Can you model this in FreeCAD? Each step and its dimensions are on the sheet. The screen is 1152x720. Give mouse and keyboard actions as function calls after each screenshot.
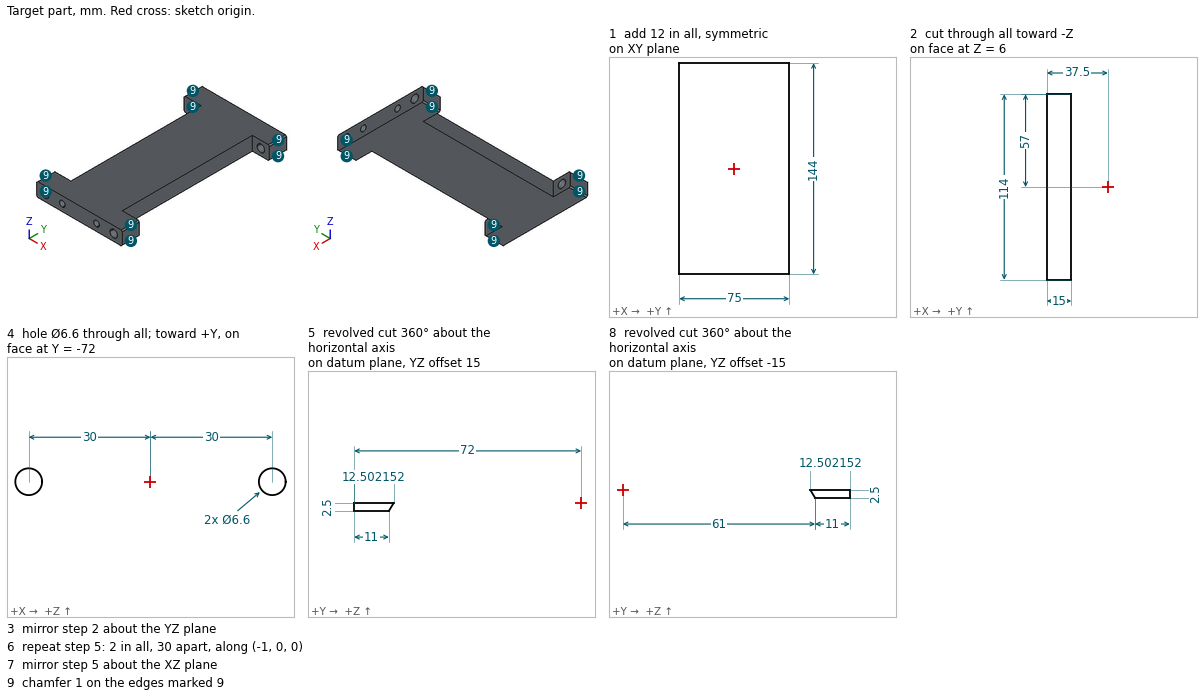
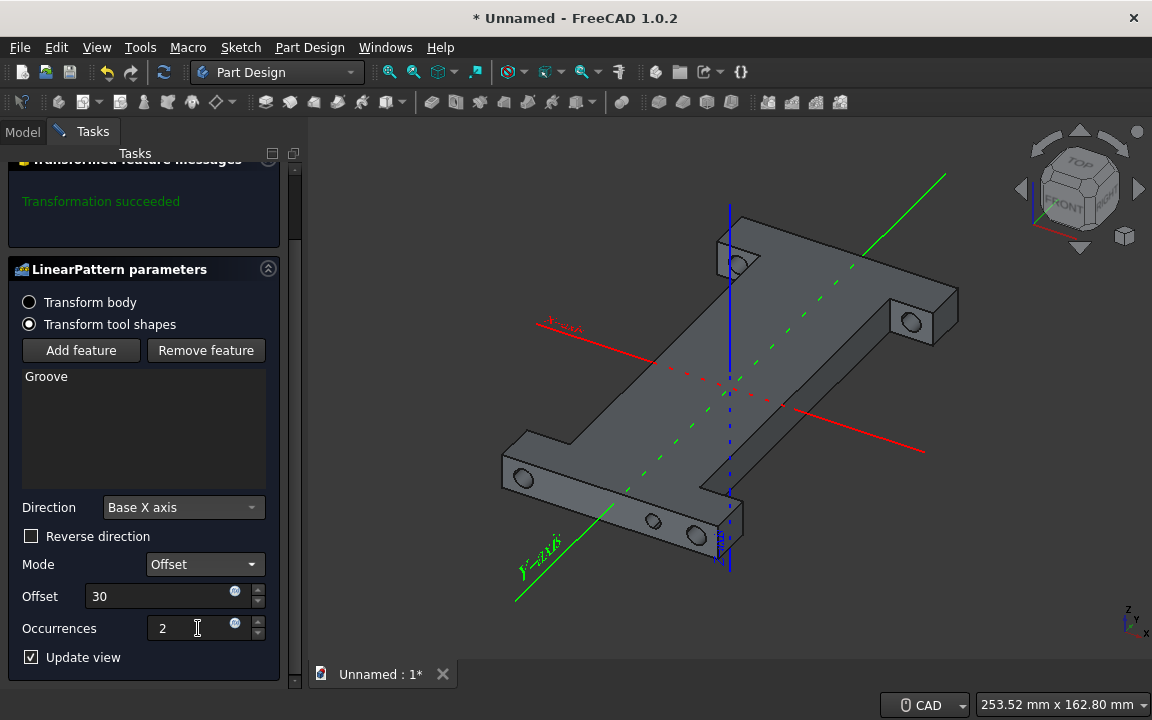
click(30, 536)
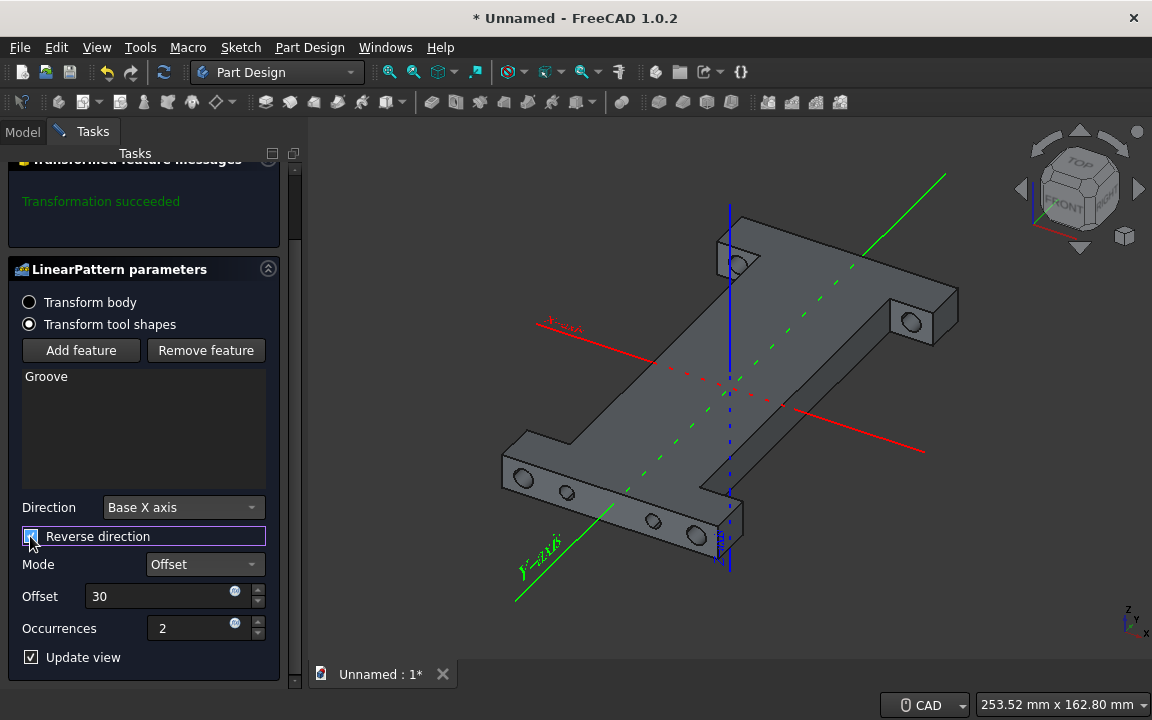
scroll(295, 426, up, 3)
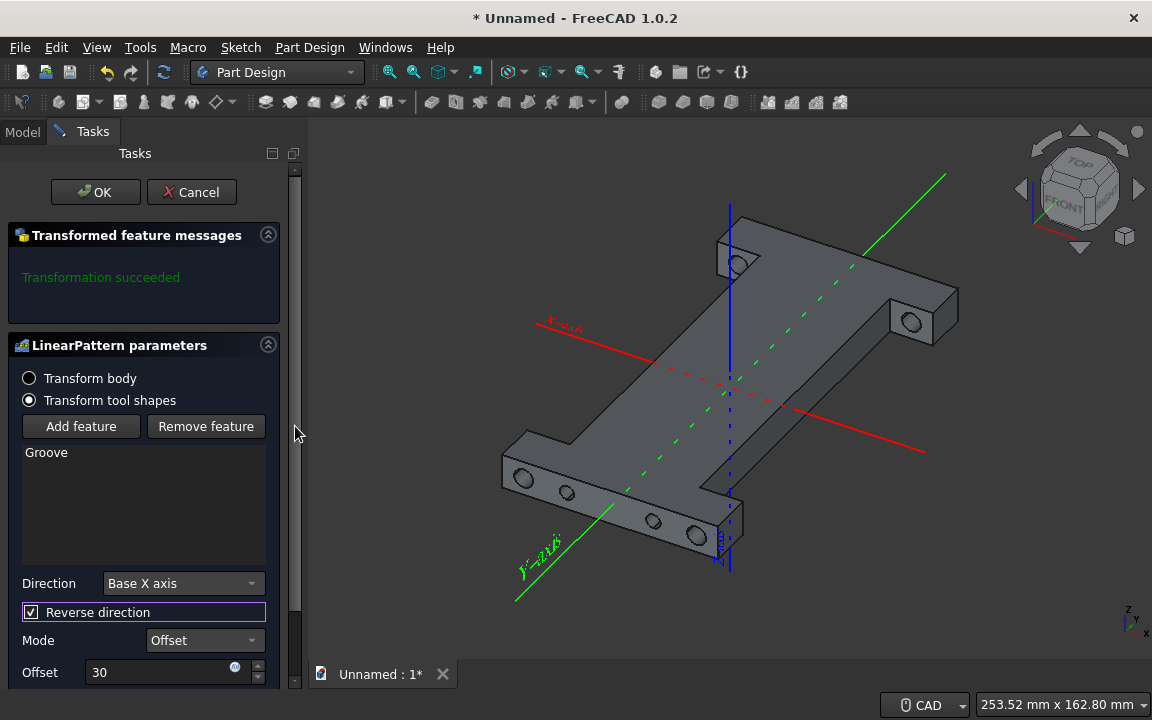
click(96, 192)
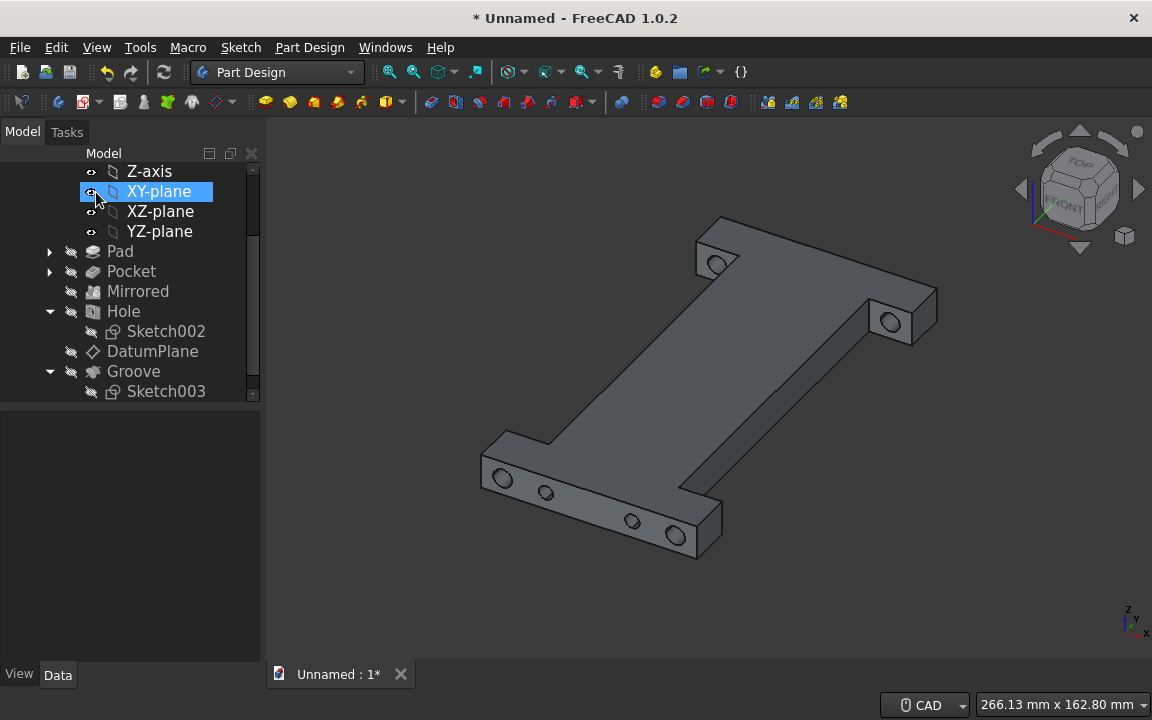
click(116, 372)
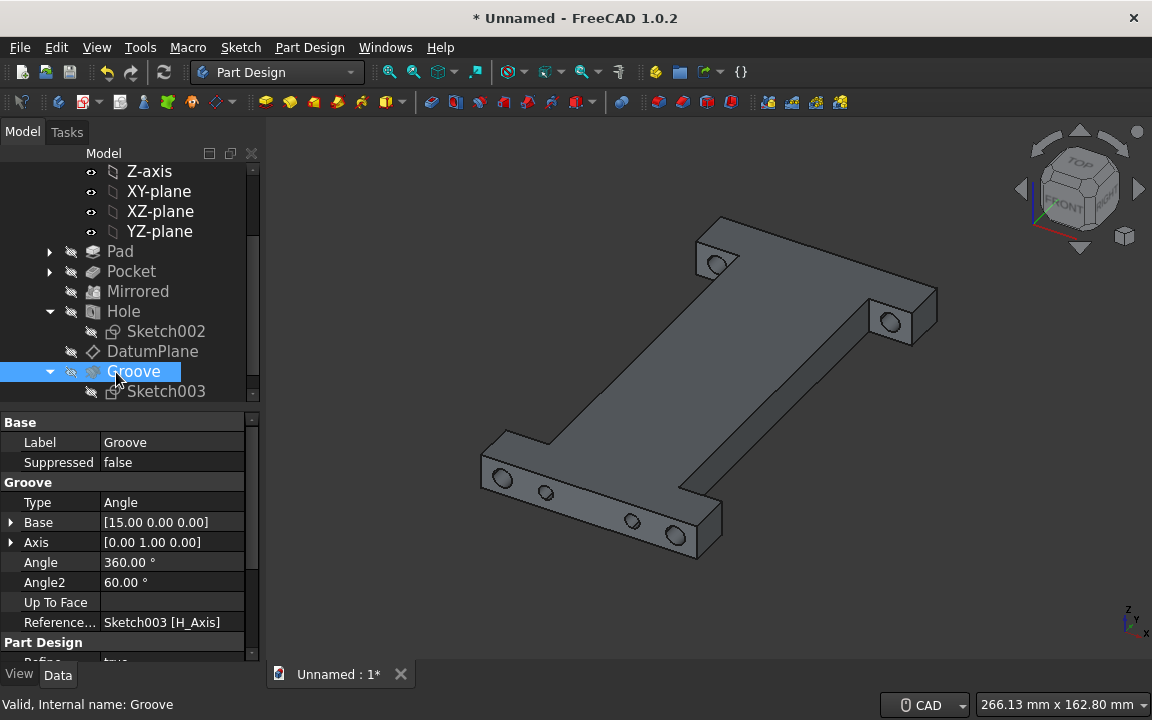
click(768, 102)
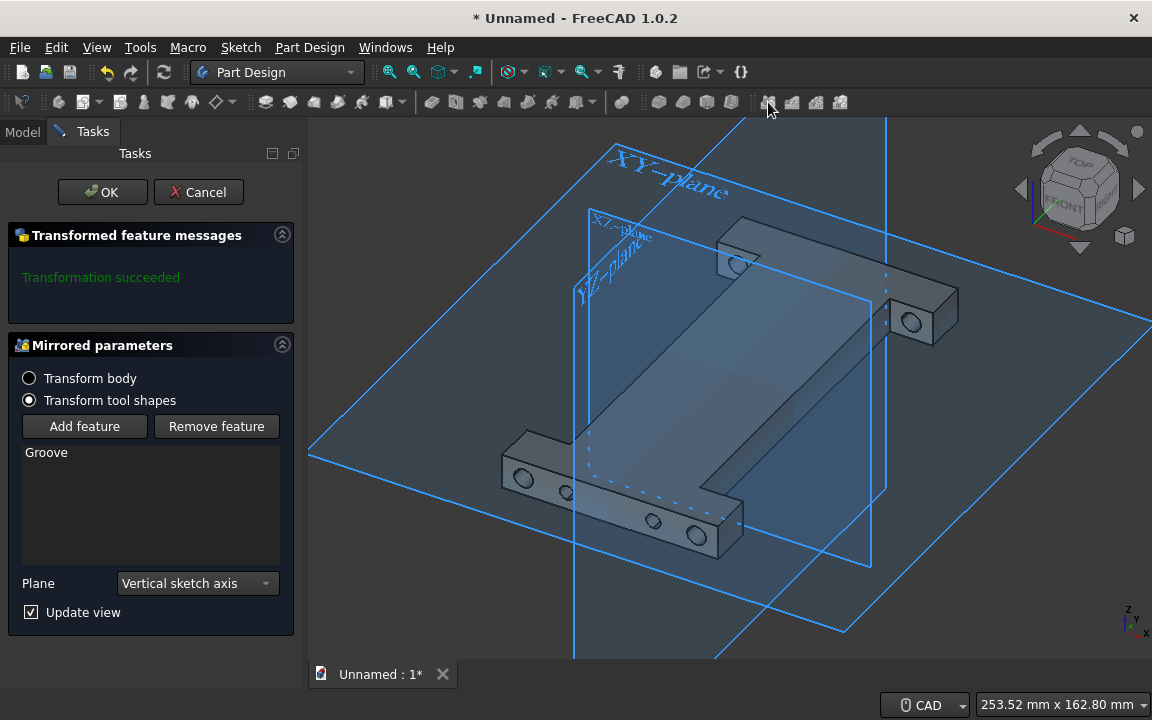
click(198, 584)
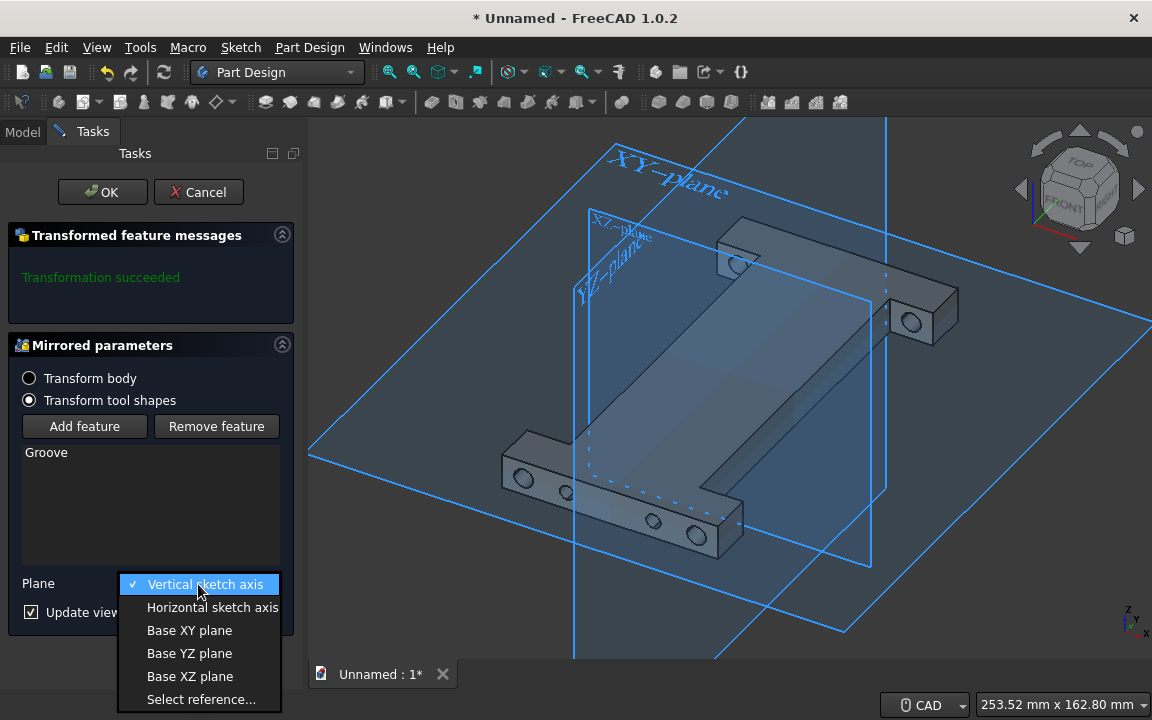
click(198, 676)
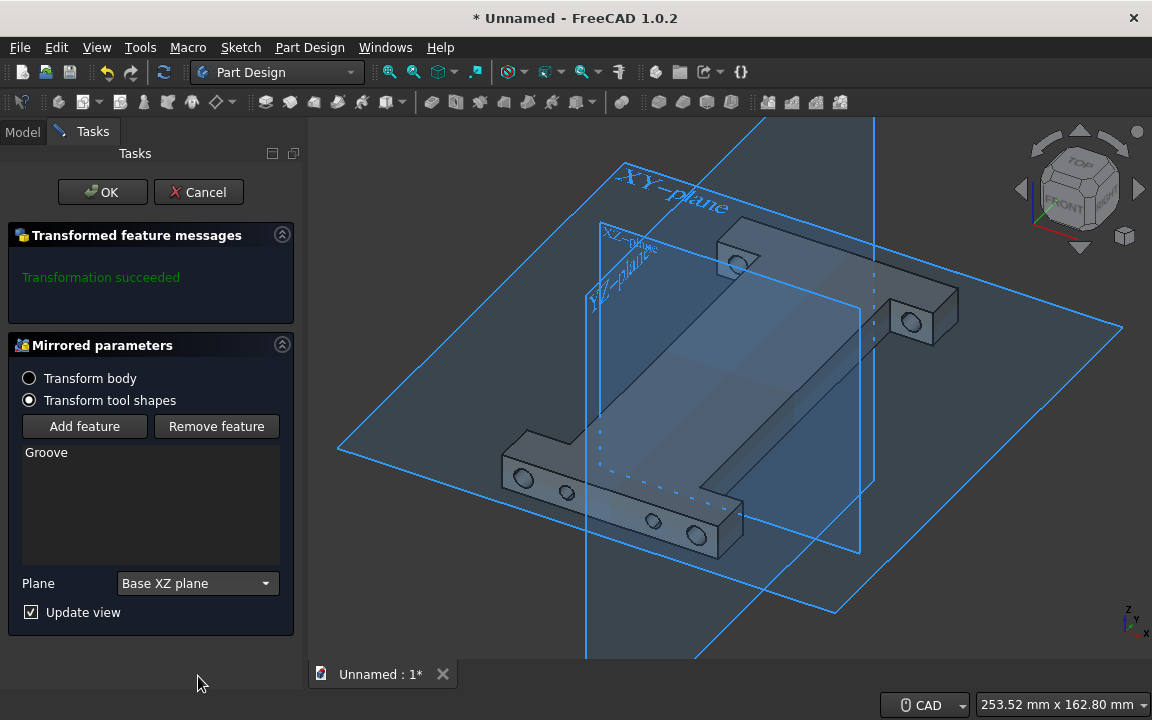
click(103, 192)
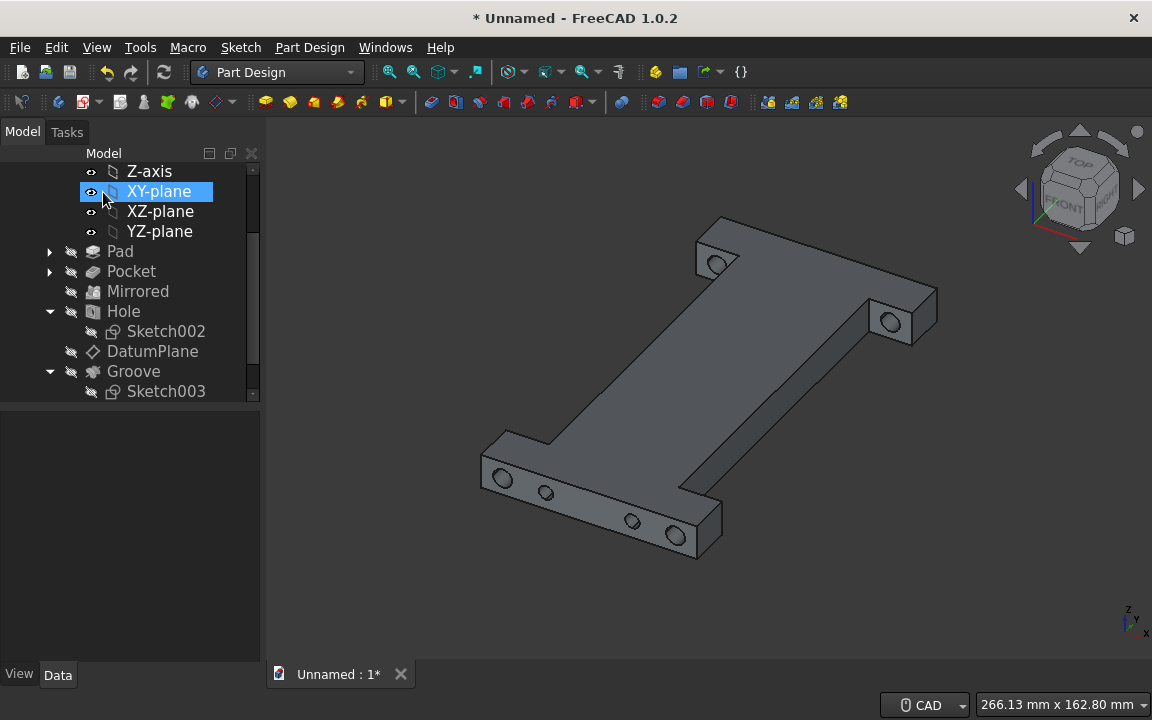
scroll(160, 287, down, 3)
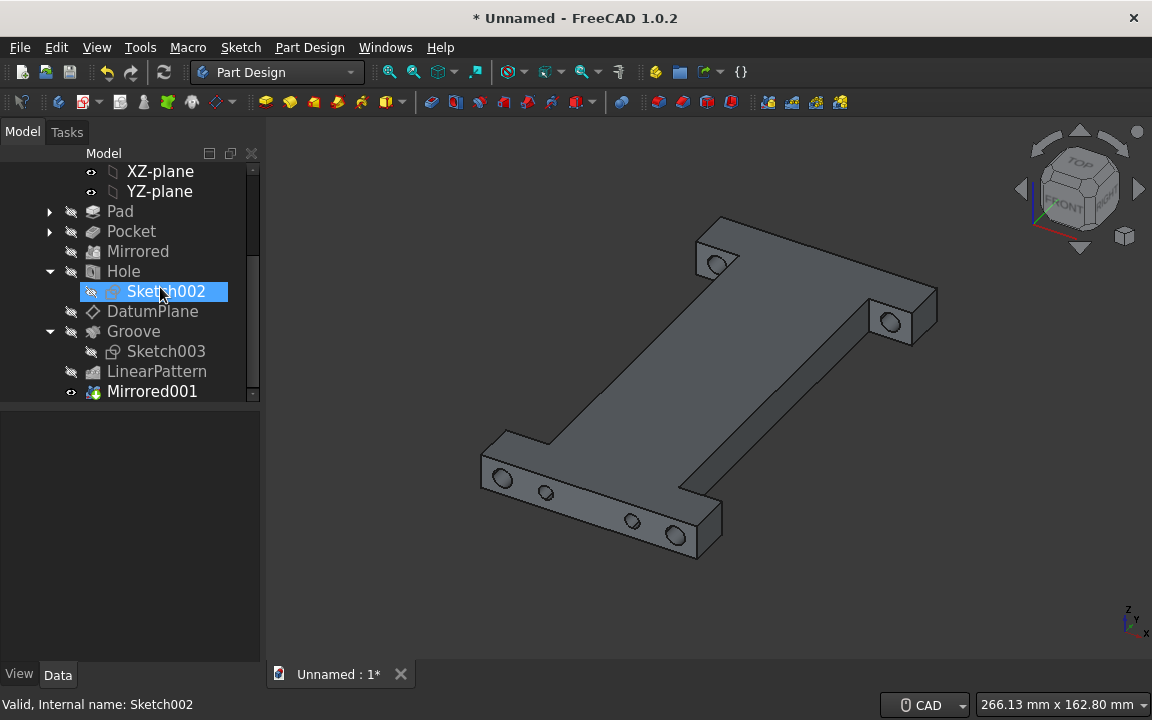
scroll(160, 287, up, 15)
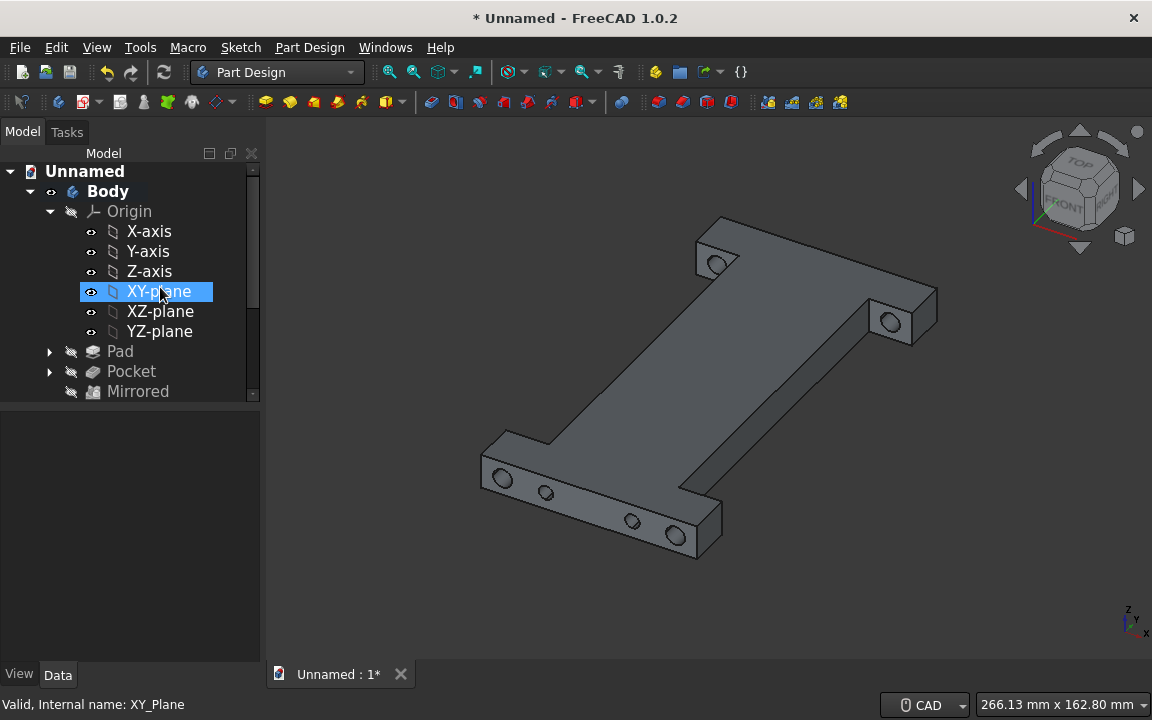
click(136, 332)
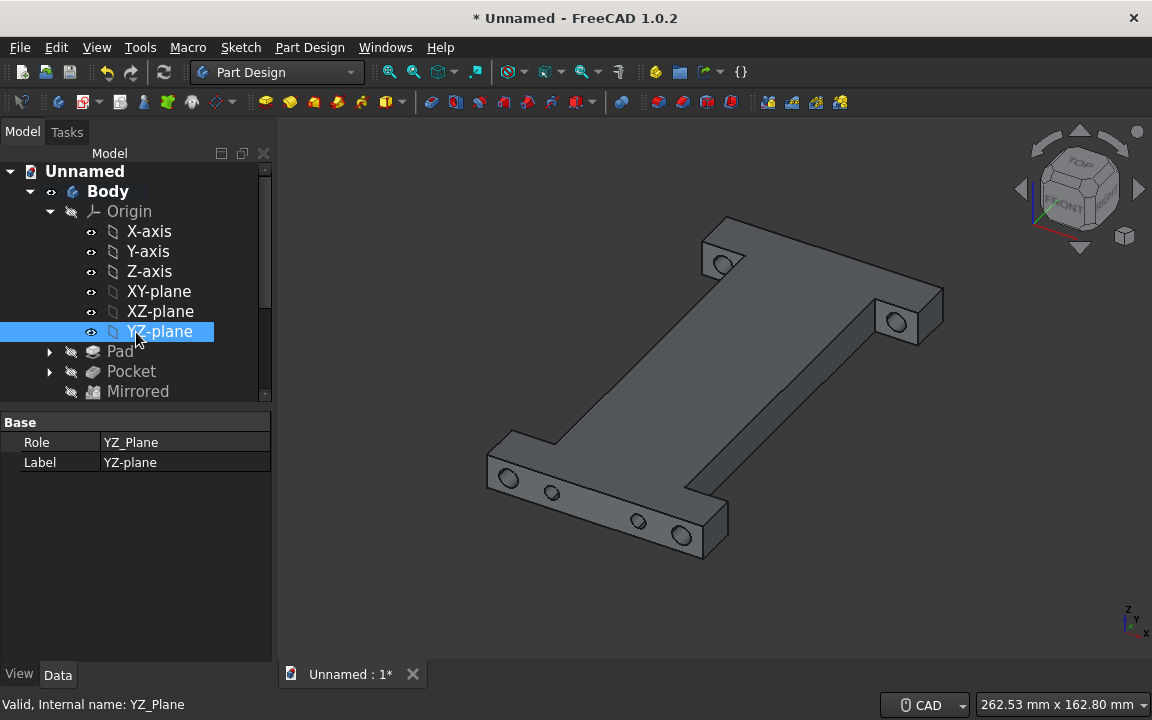
click(216, 102)